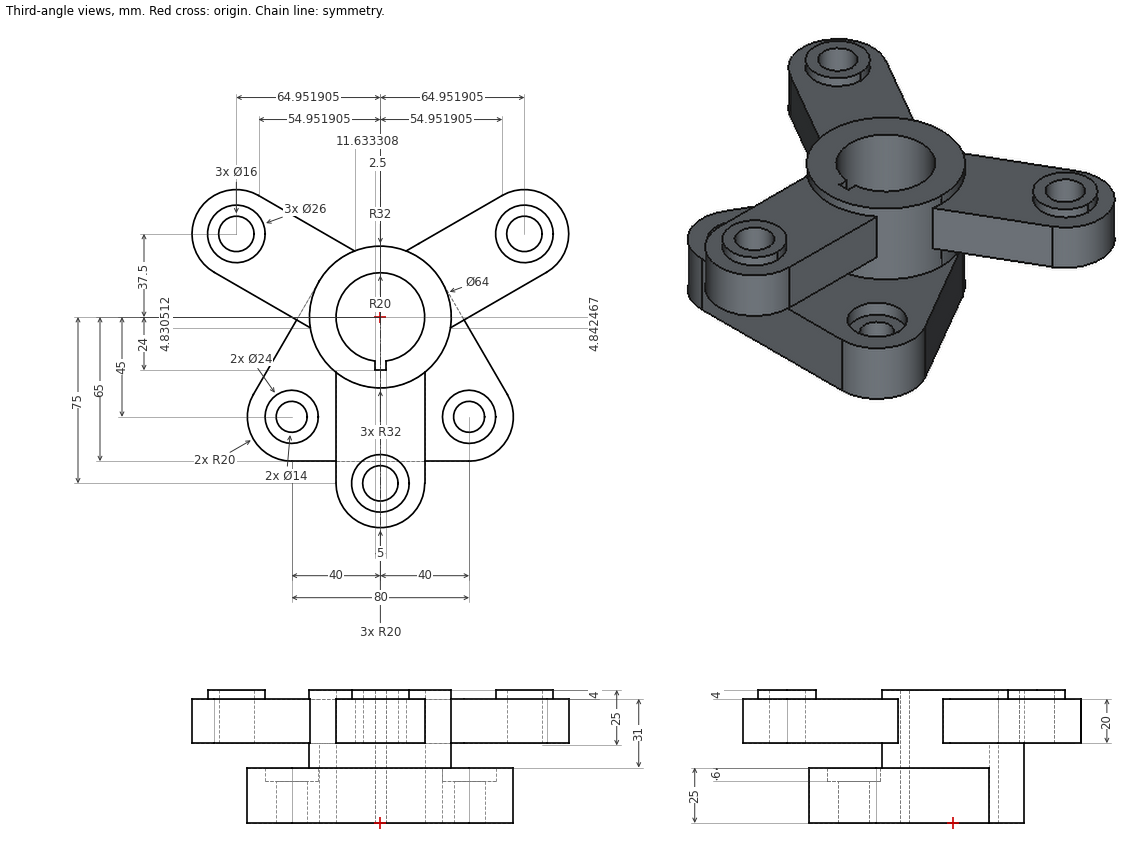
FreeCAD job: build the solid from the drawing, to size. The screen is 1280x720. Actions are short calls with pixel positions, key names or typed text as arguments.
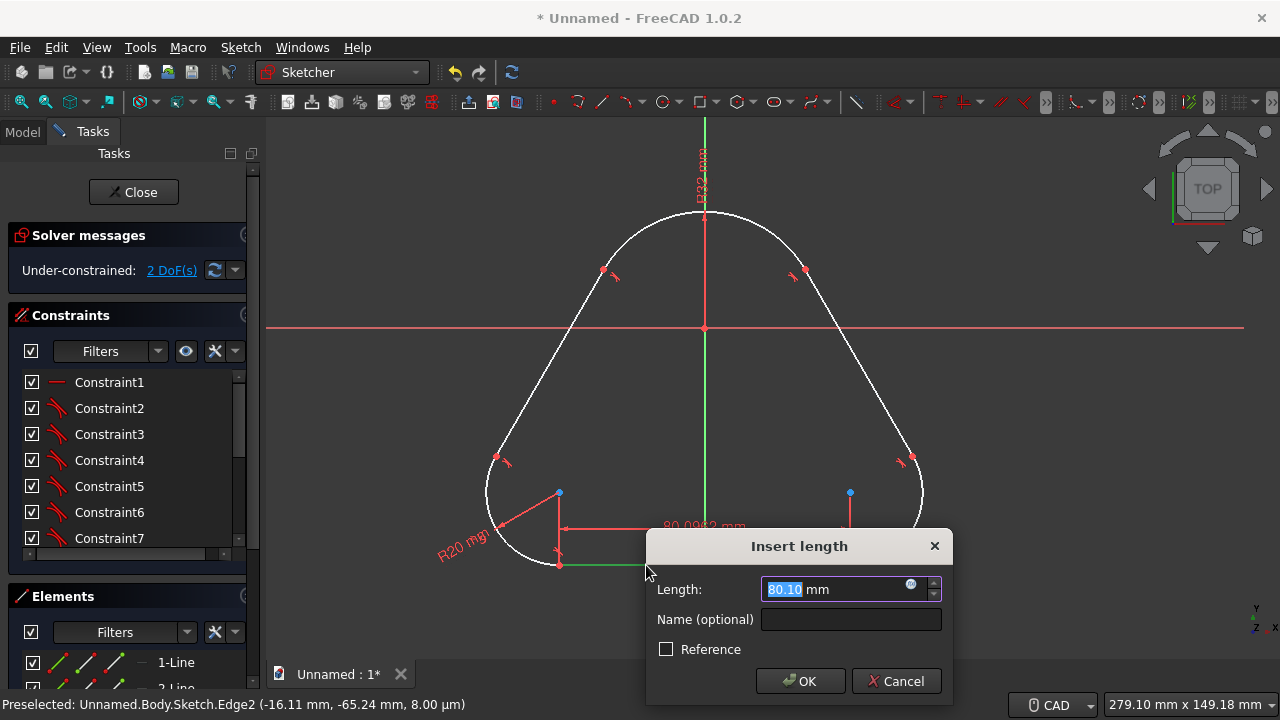
text(80)
key(Return)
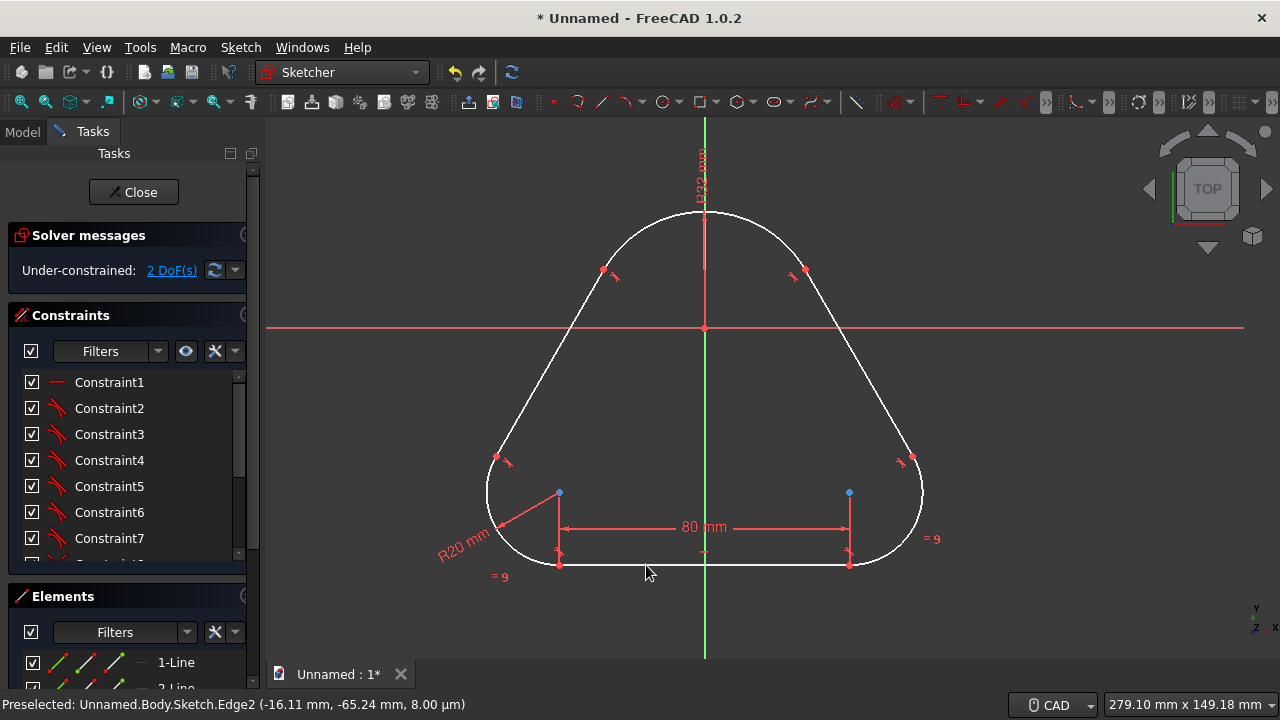
click(559, 565)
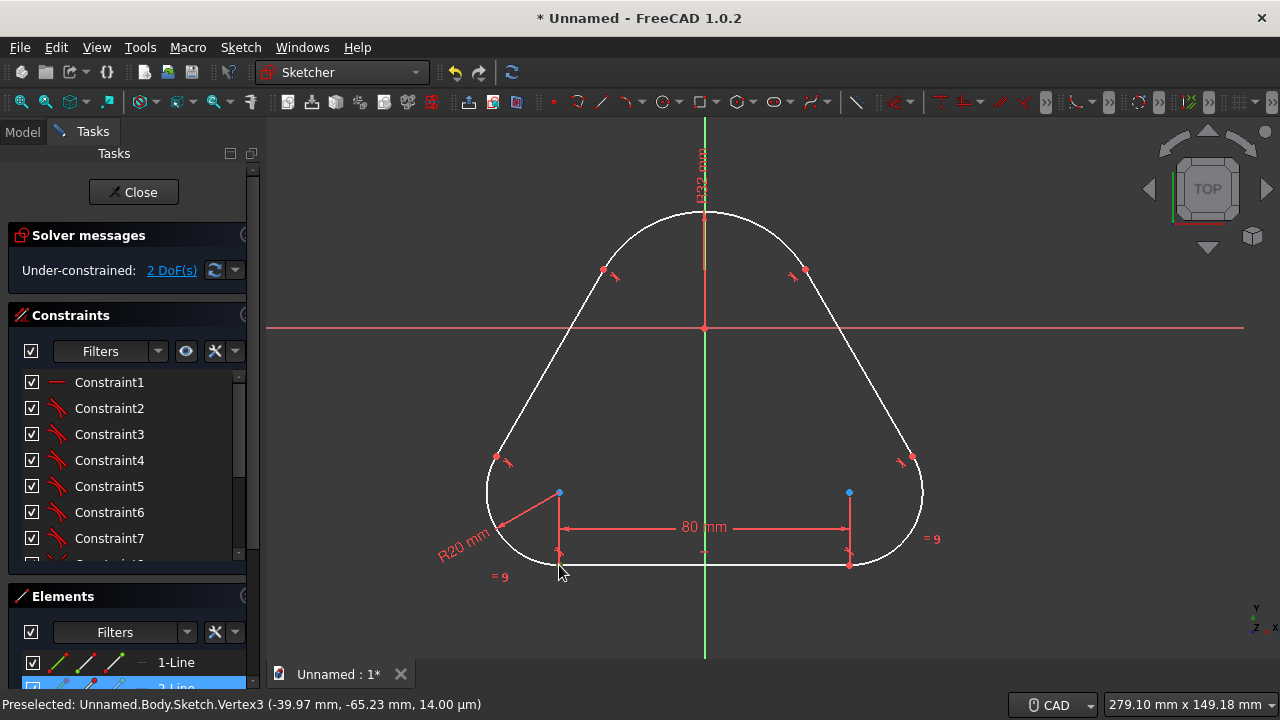
key(l)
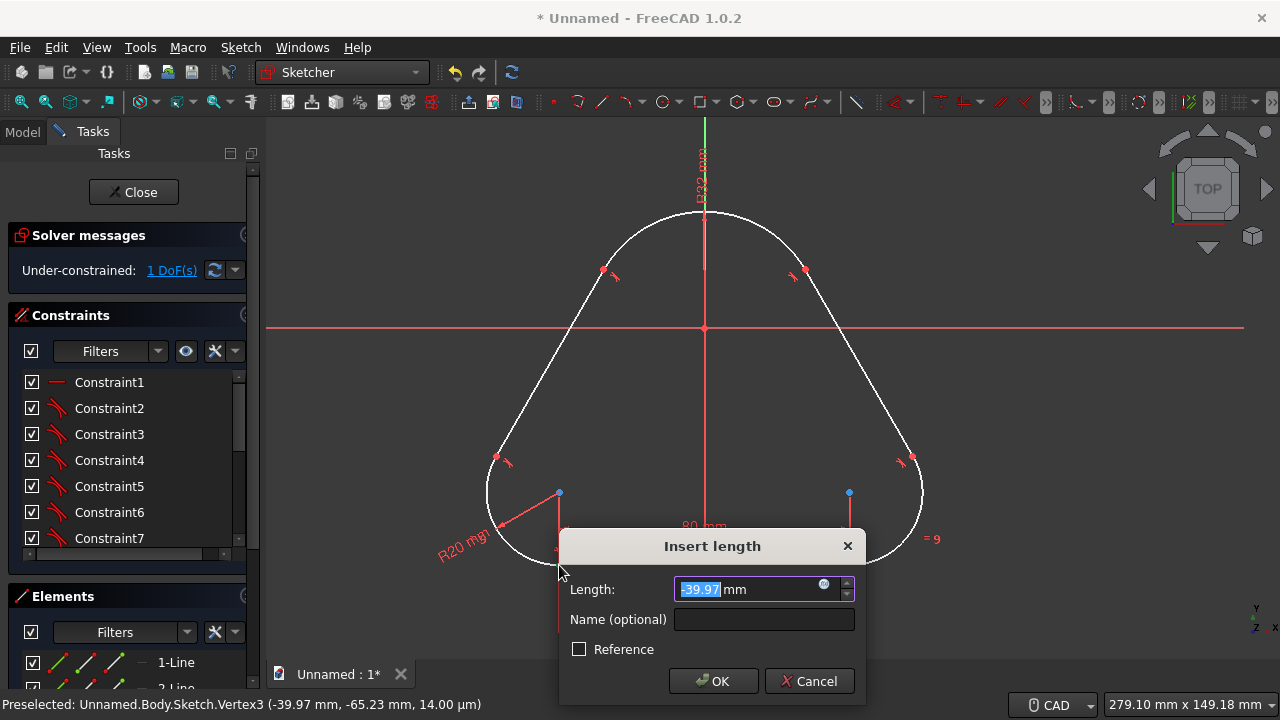
text(-40)
key(Return)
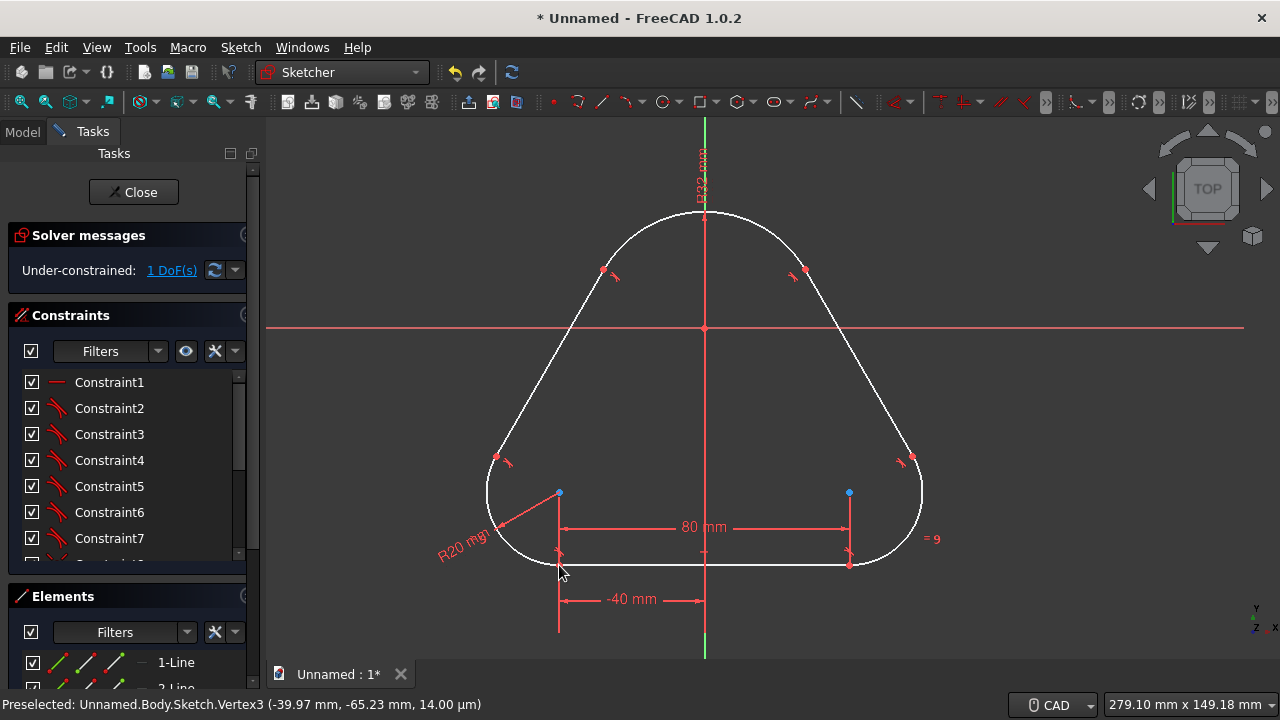
click(559, 565)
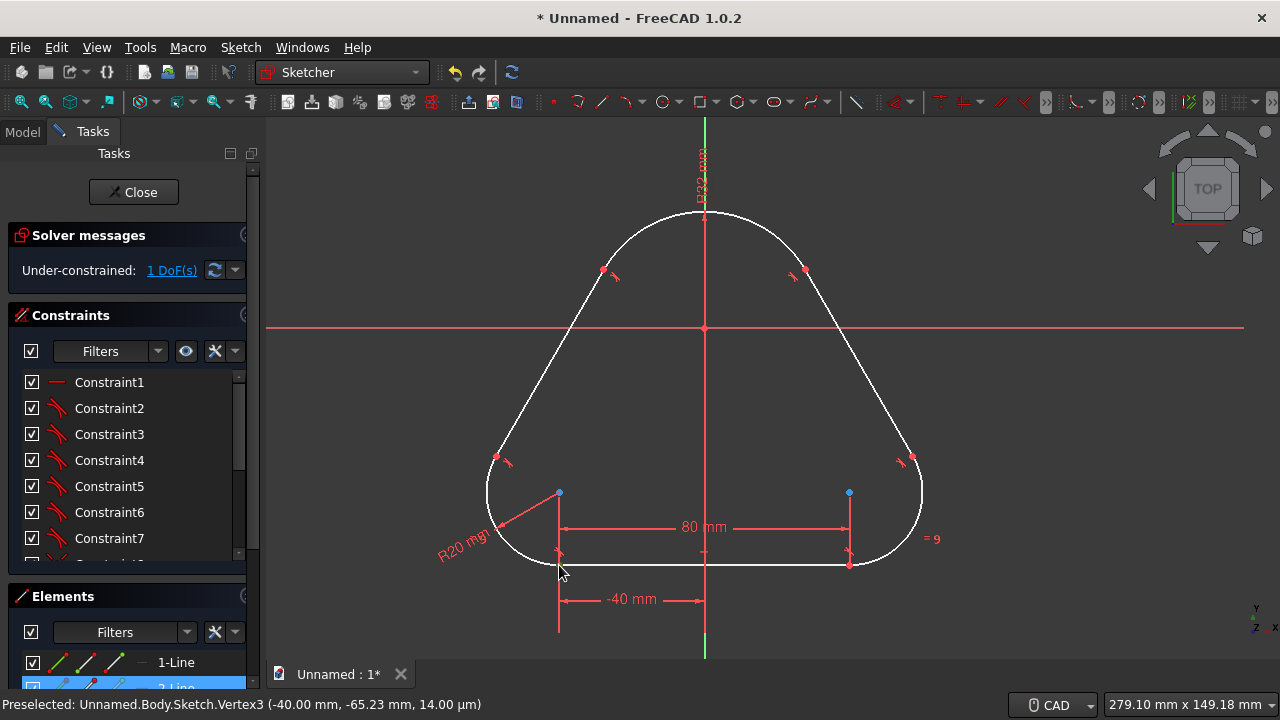
key(i)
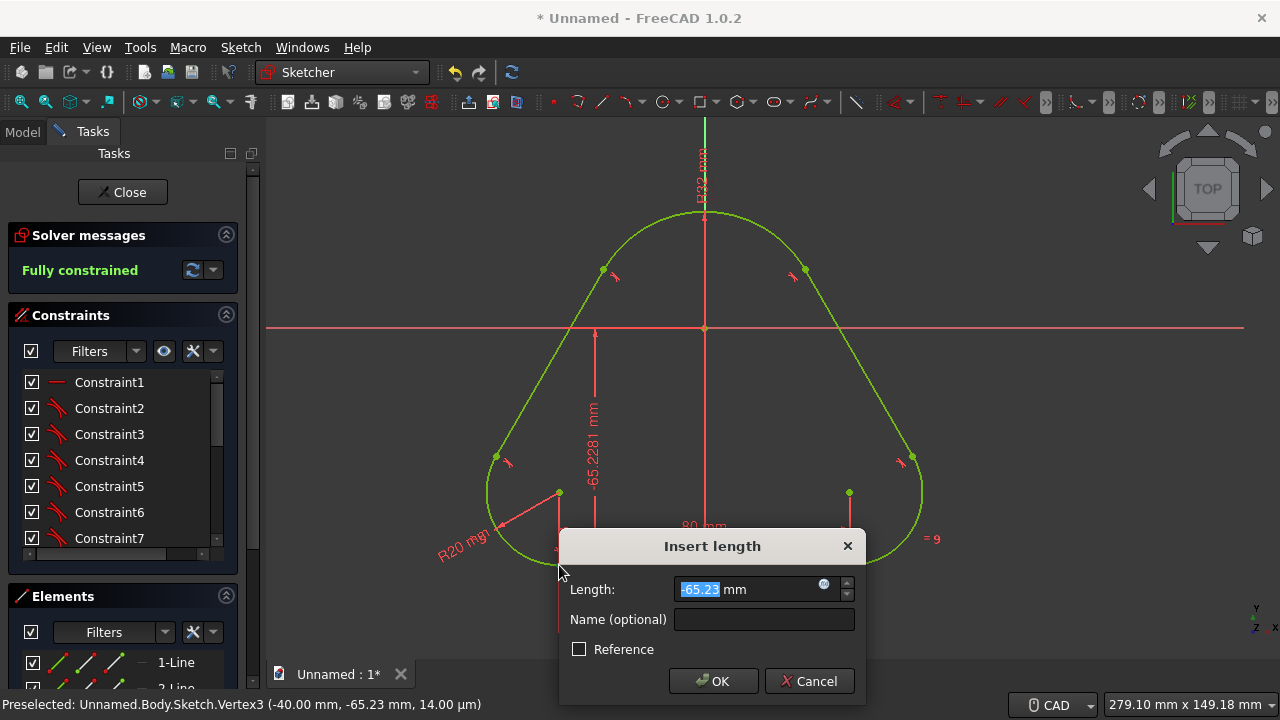
text(-65)
key(Return)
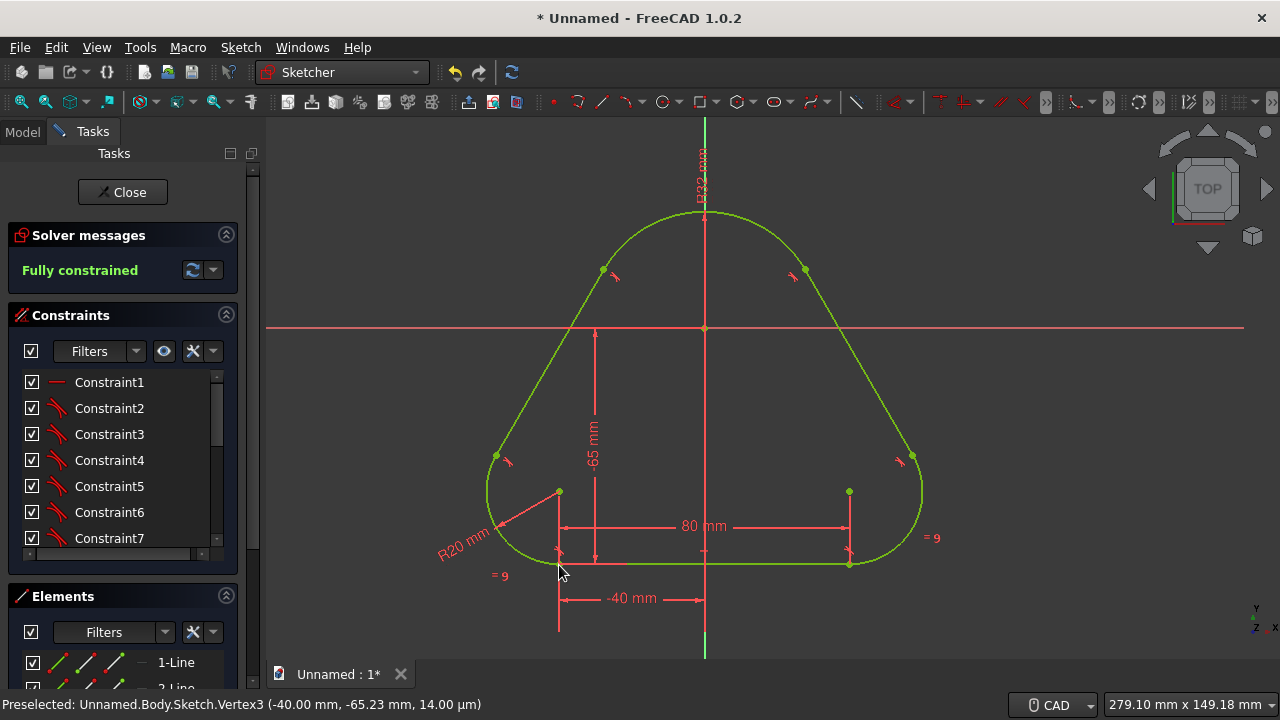
click(123, 192)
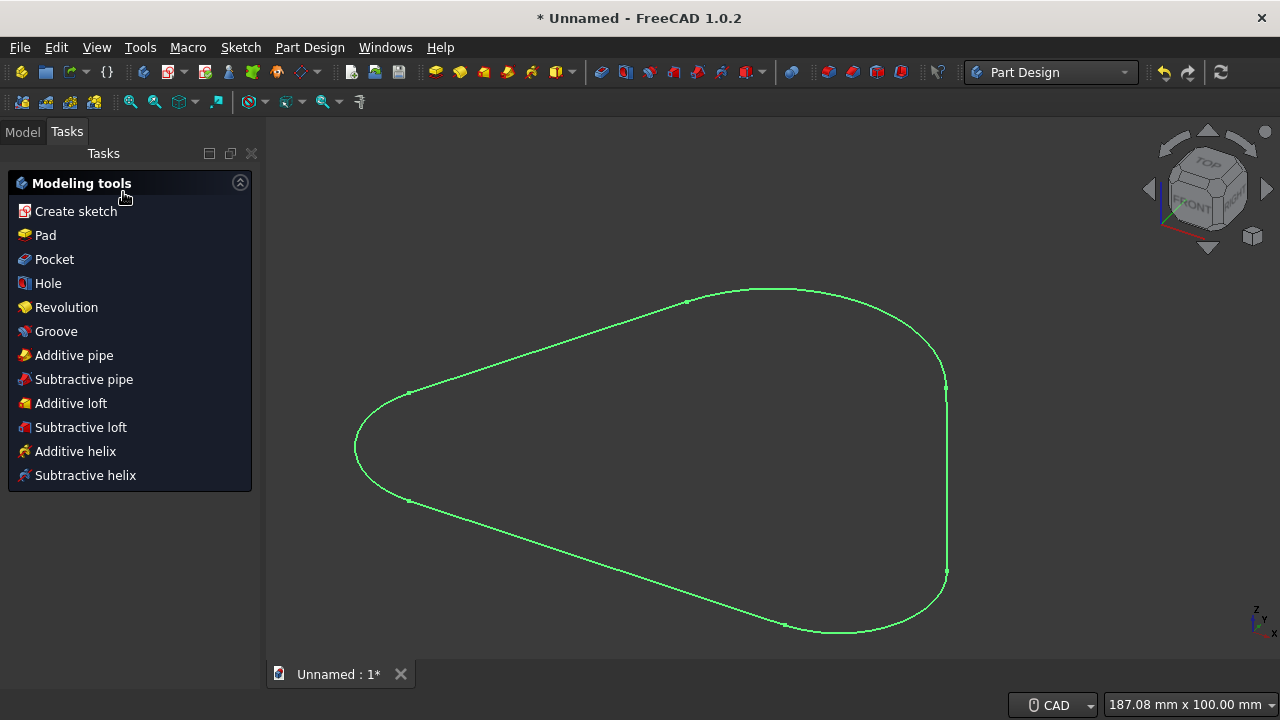
click(436, 72)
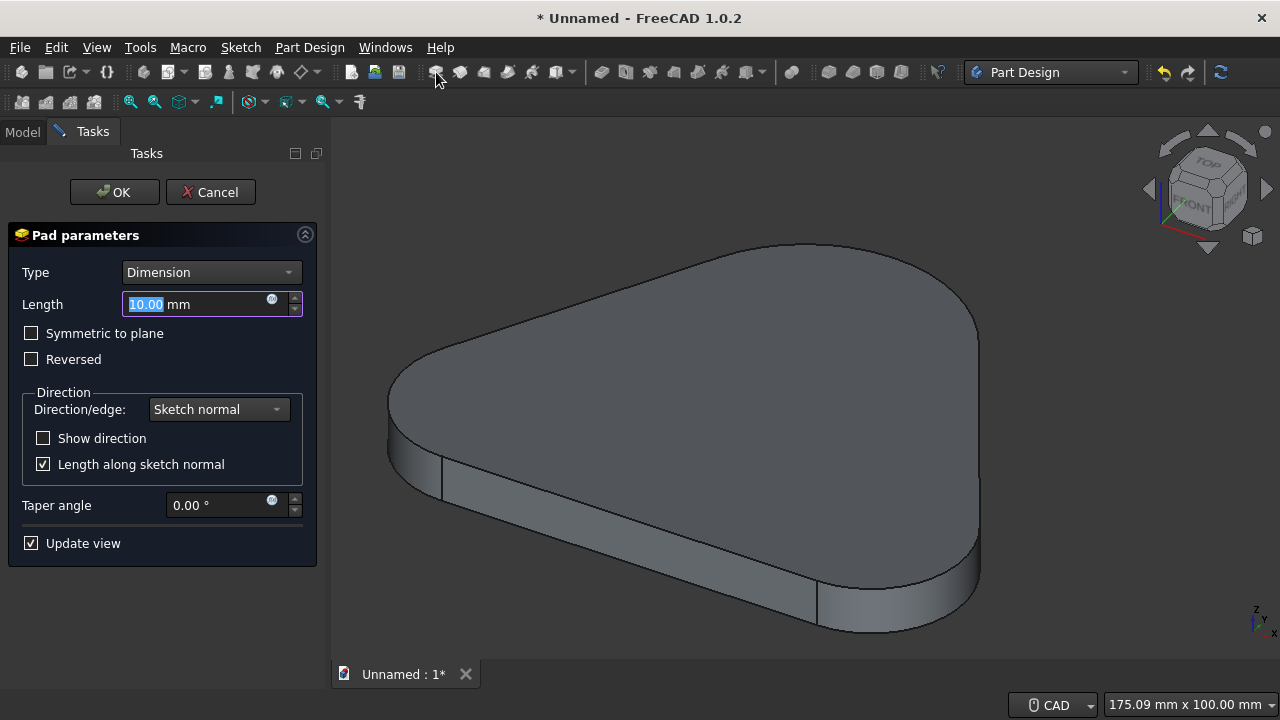
text(25)
key(Tab)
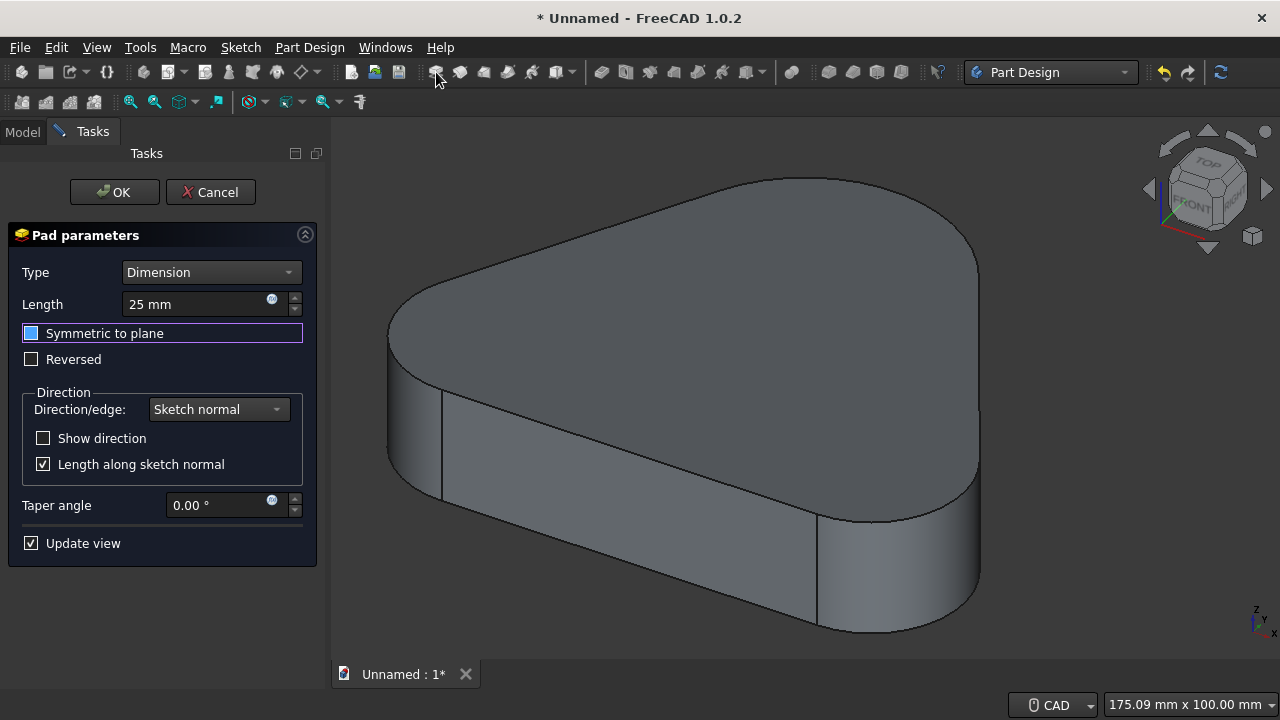
click(115, 192)